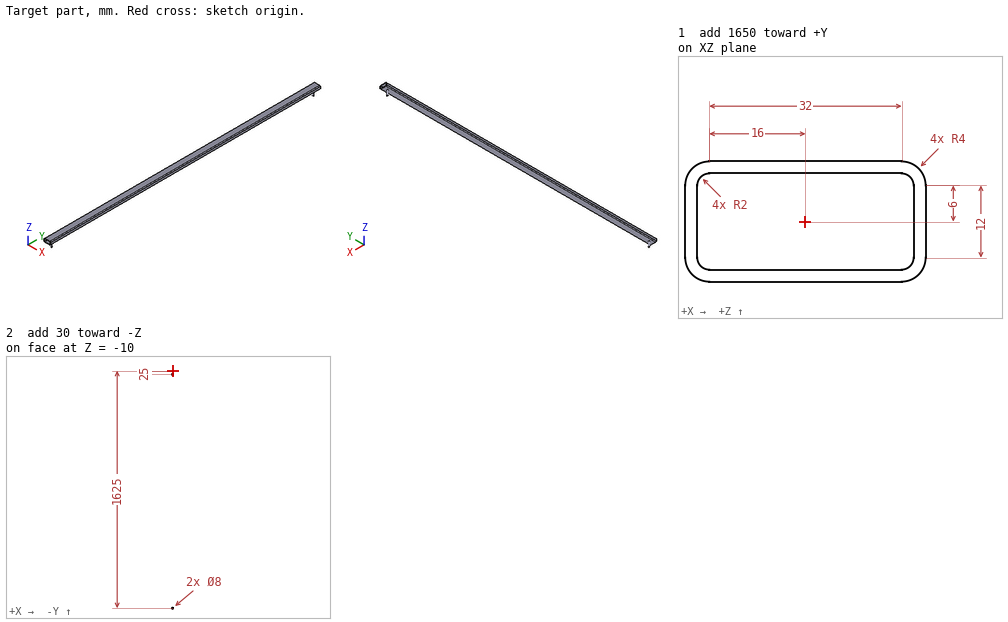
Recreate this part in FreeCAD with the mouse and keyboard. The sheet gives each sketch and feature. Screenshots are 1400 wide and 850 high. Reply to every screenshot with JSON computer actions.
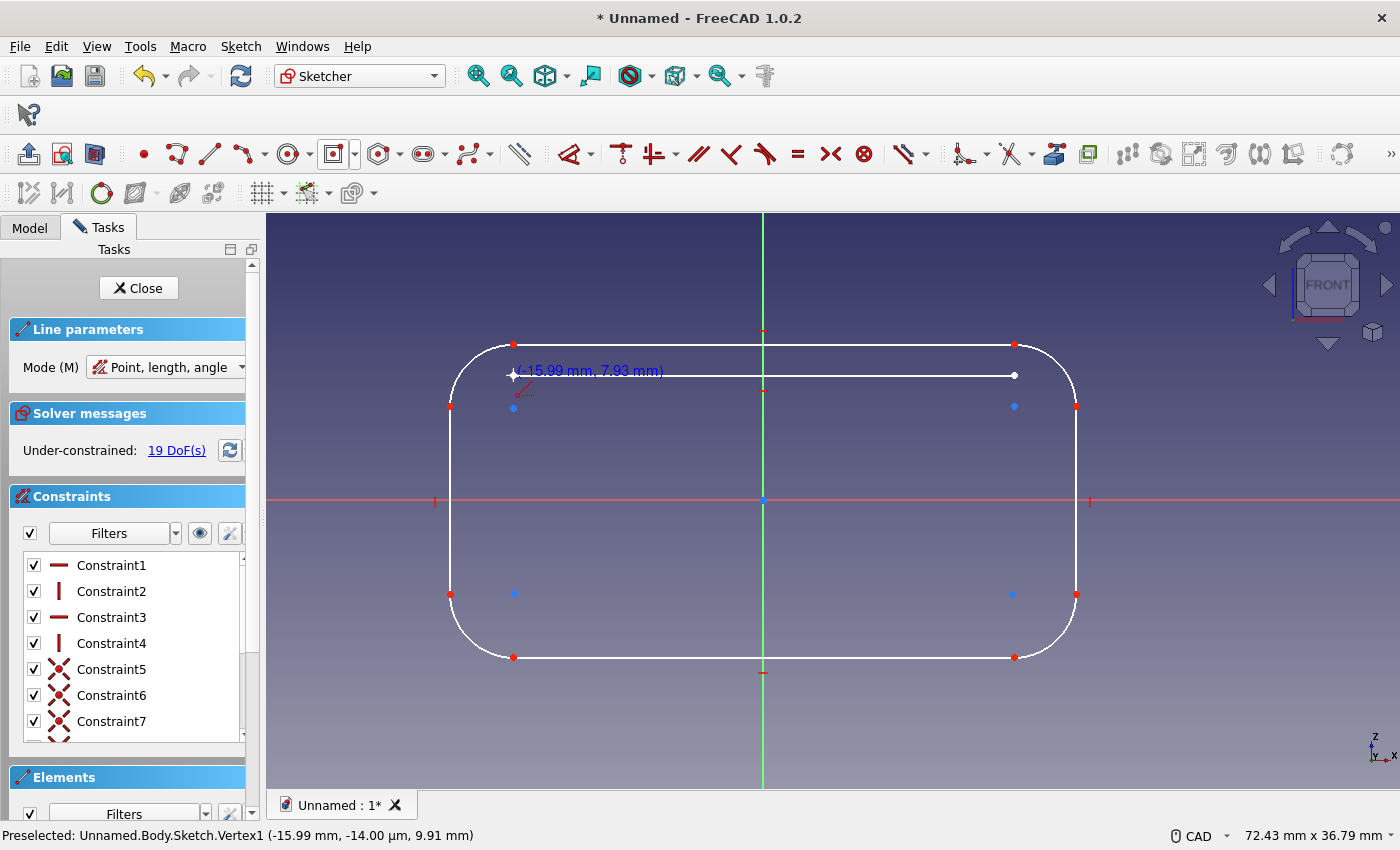
{"action": "left_click", "coordinate": [482, 406]}
{"action": "left_click", "coordinate": [482, 594]}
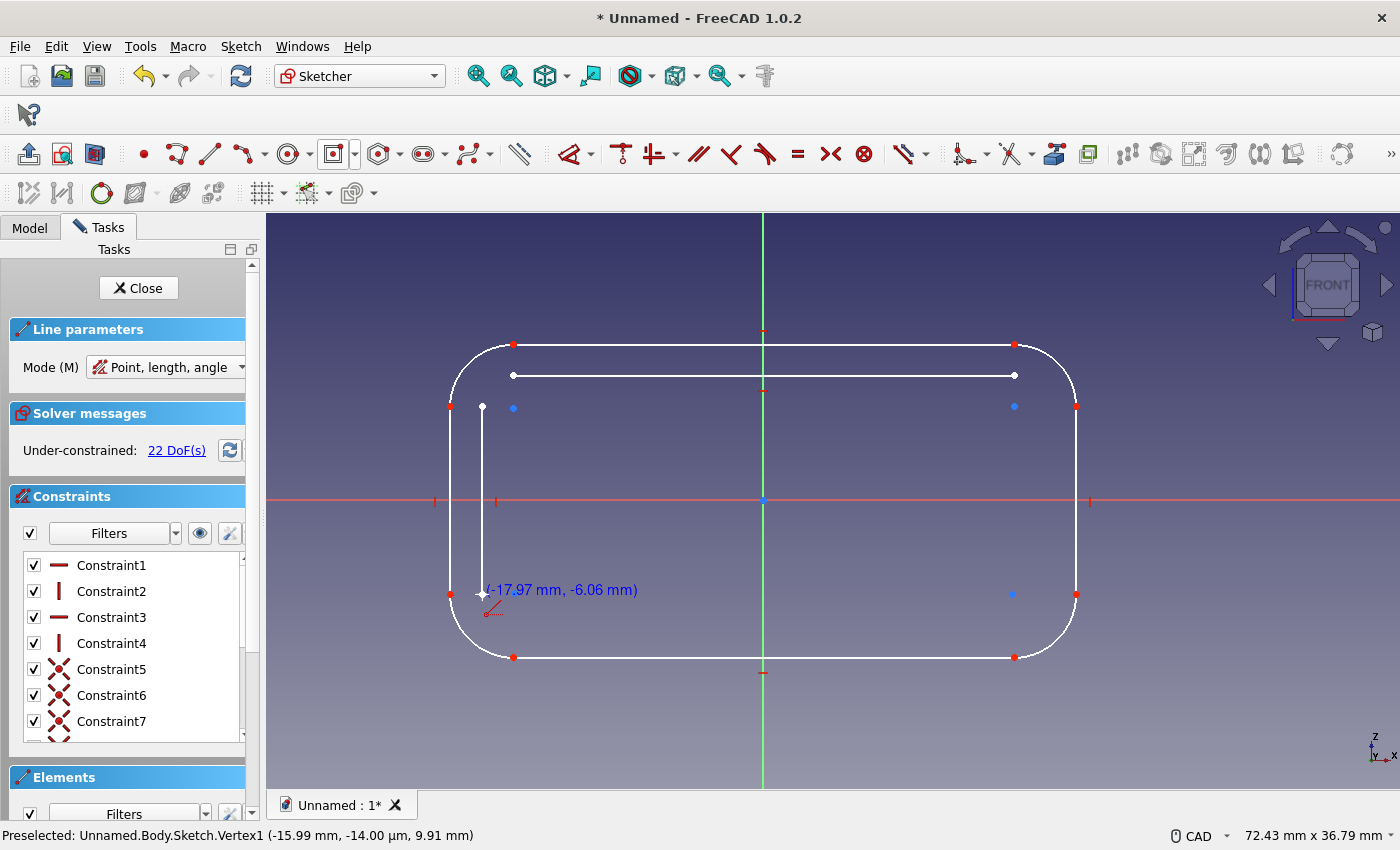
{"action": "left_click", "coordinate": [513, 625]}
{"action": "left_click", "coordinate": [1014, 625]}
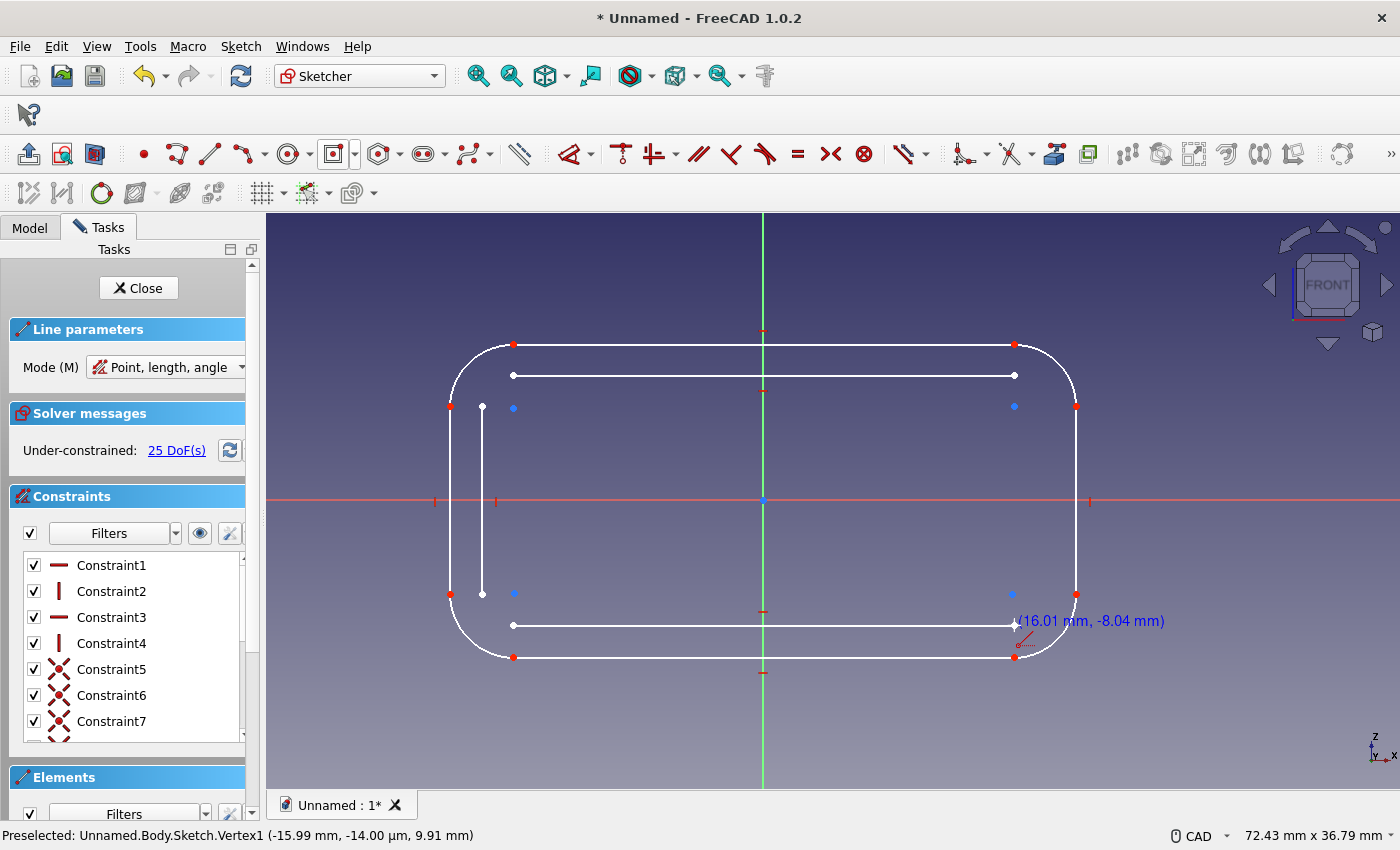
{"action": "left_click", "coordinate": [1045, 594]}
{"action": "left_click", "coordinate": [1045, 406]}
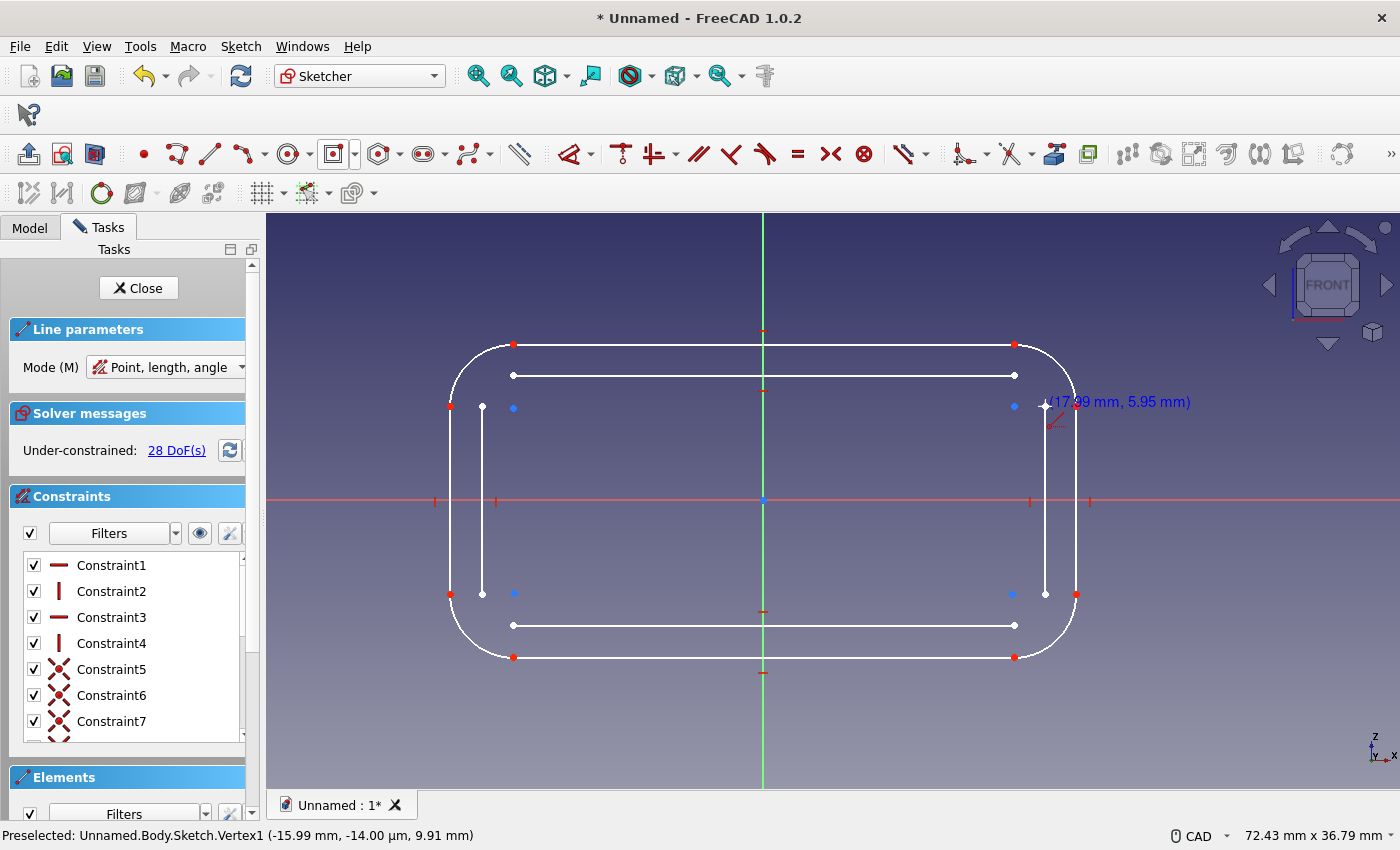
{"action": "left_click", "coordinate": [242, 154]}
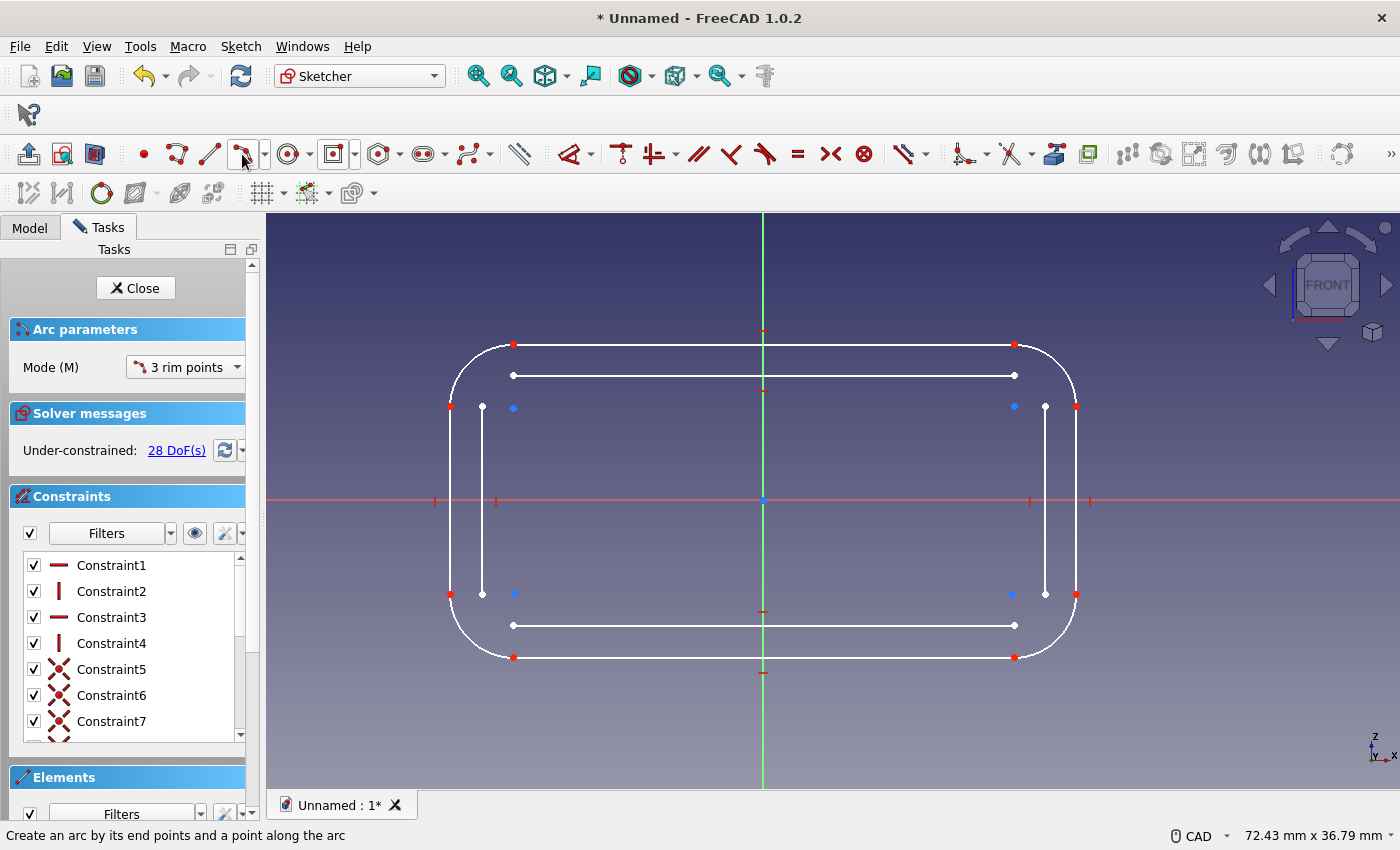
{"action": "left_click", "coordinate": [513, 376]}
{"action": "left_click", "coordinate": [482, 407]}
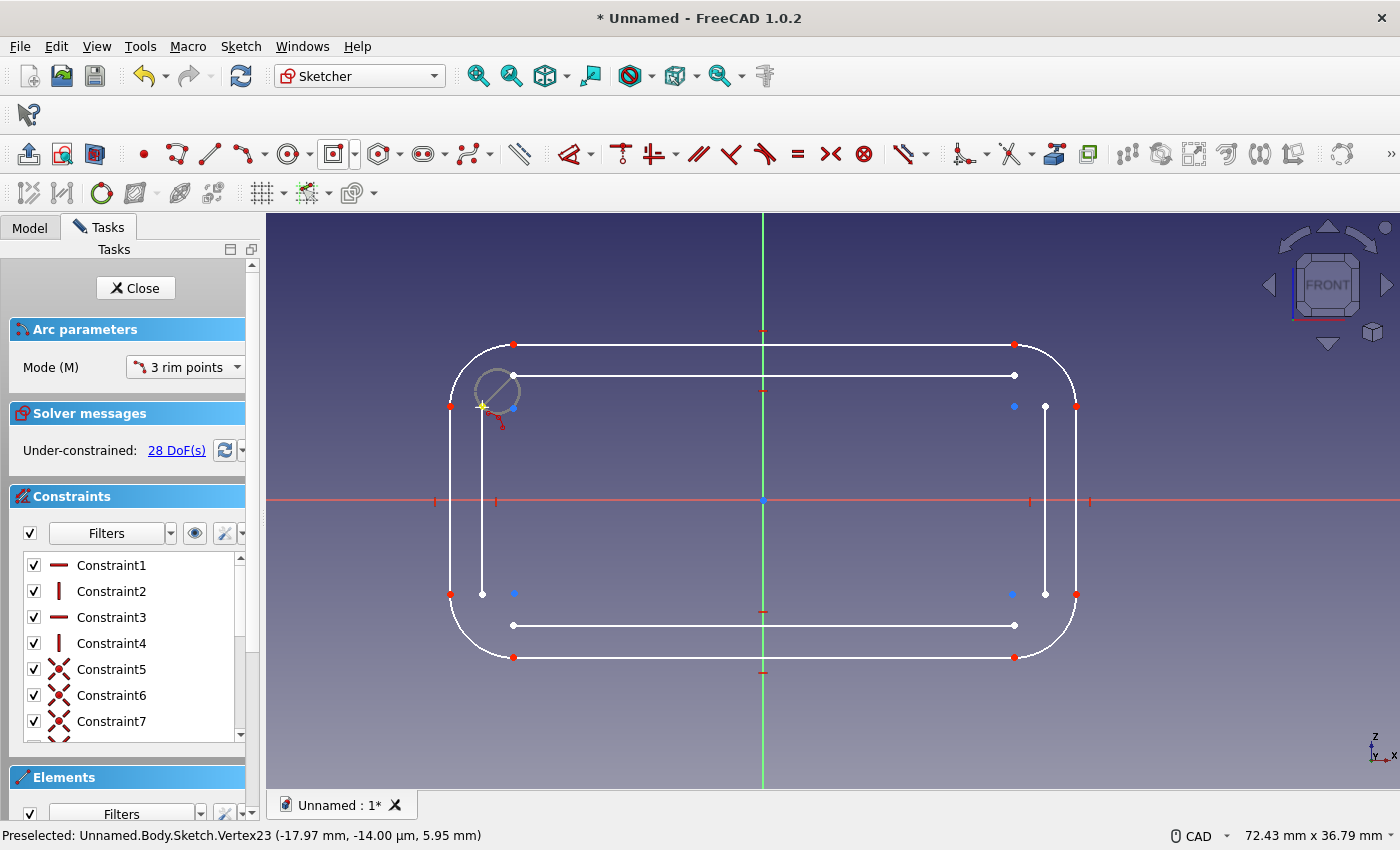
{"action": "scroll", "coordinate": [491, 384], "scroll_direction": "up", "scroll_amount": 3}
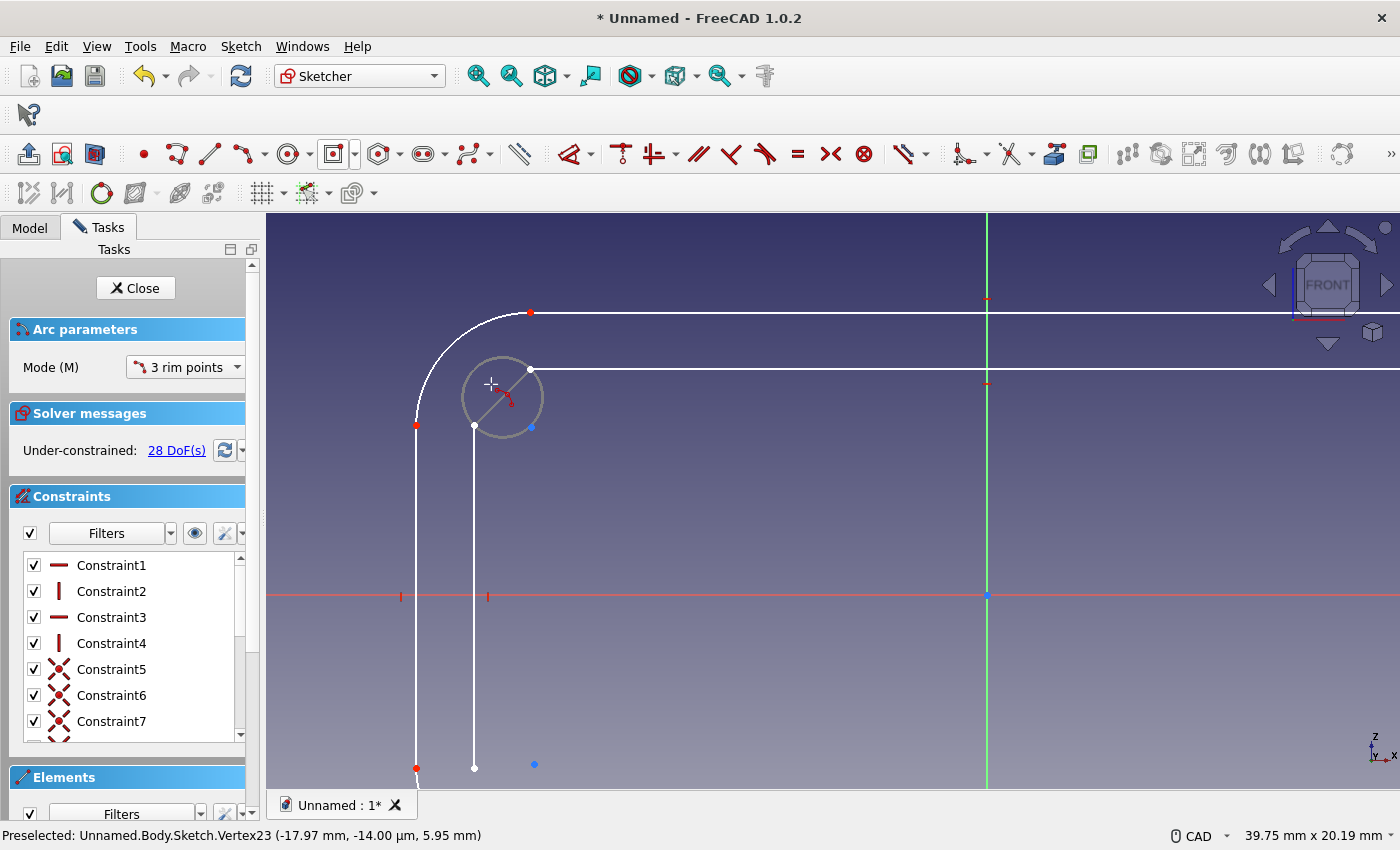
{"action": "left_click", "coordinate": [490, 384]}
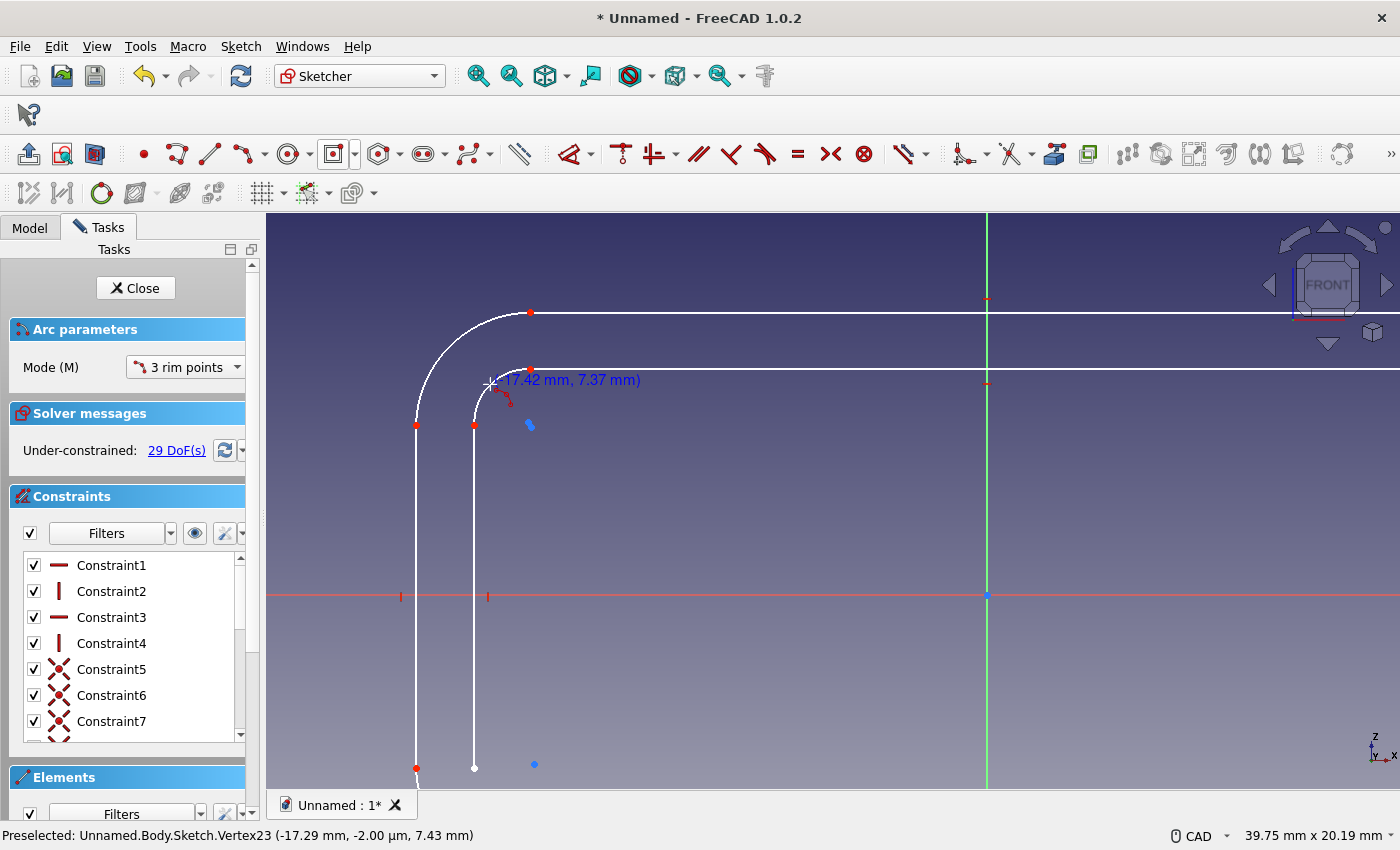
{"action": "scroll", "coordinate": [494, 386], "scroll_direction": "down", "scroll_amount": 3}